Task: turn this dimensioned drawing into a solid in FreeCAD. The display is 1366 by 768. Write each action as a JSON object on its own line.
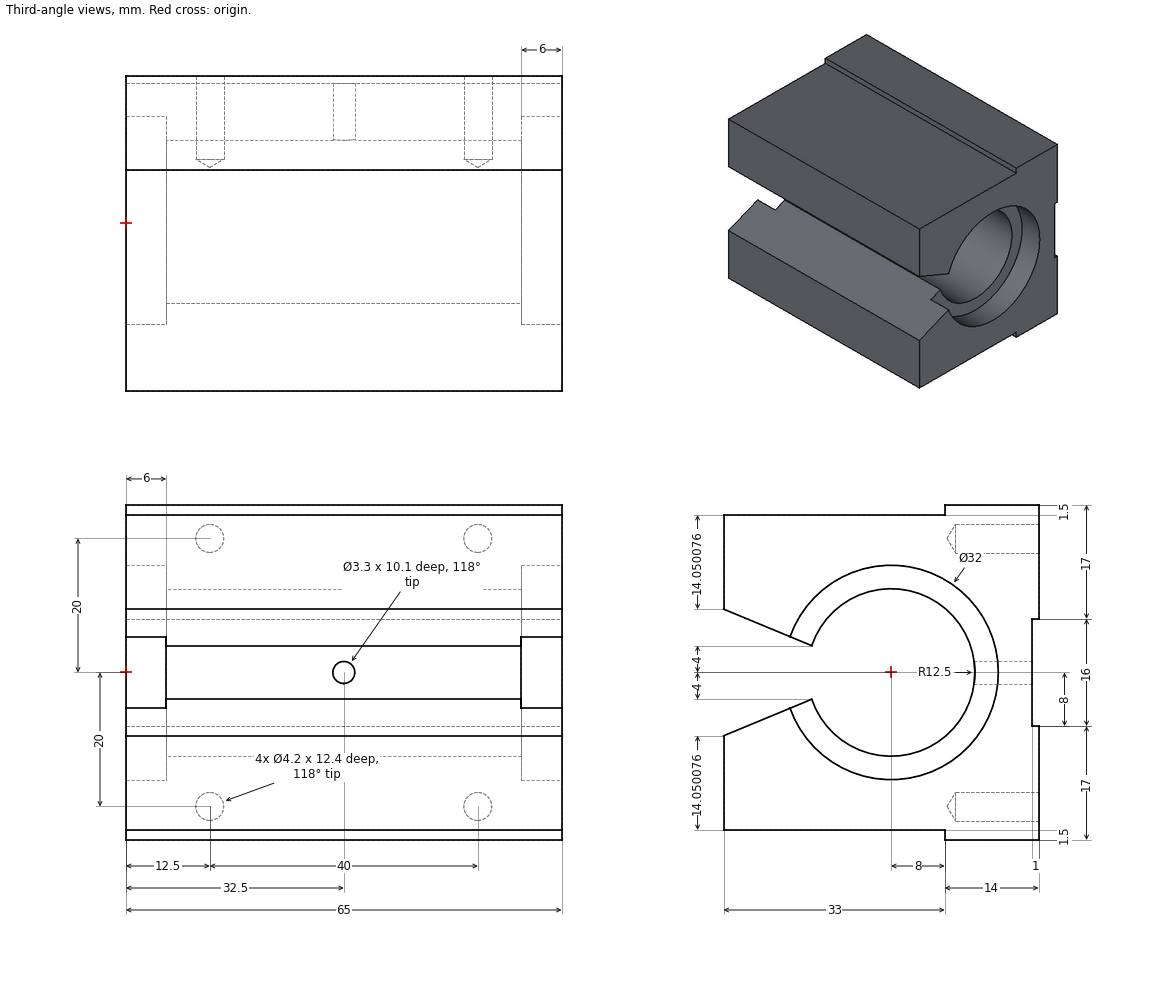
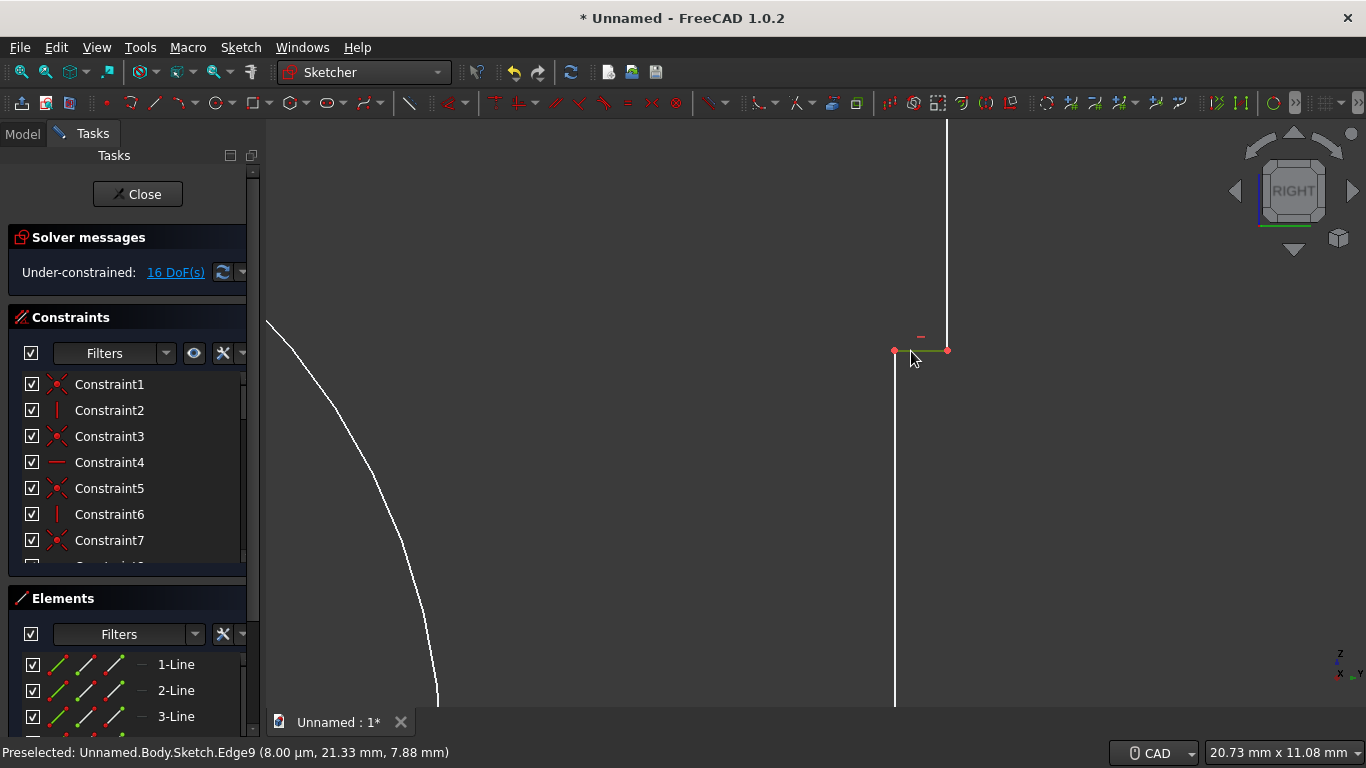
{"action": "key", "text": "l"}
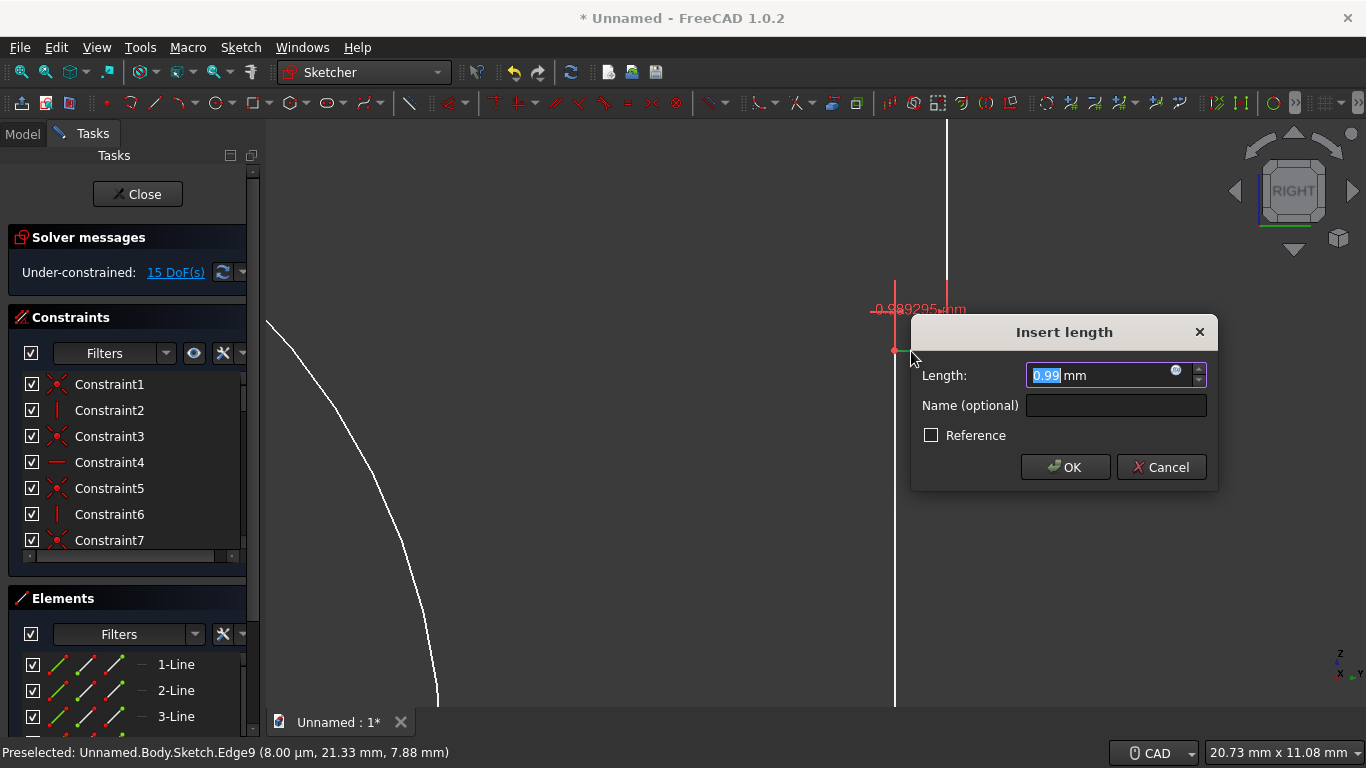
{"action": "type", "text": "1"}
{"action": "key", "text": "Return"}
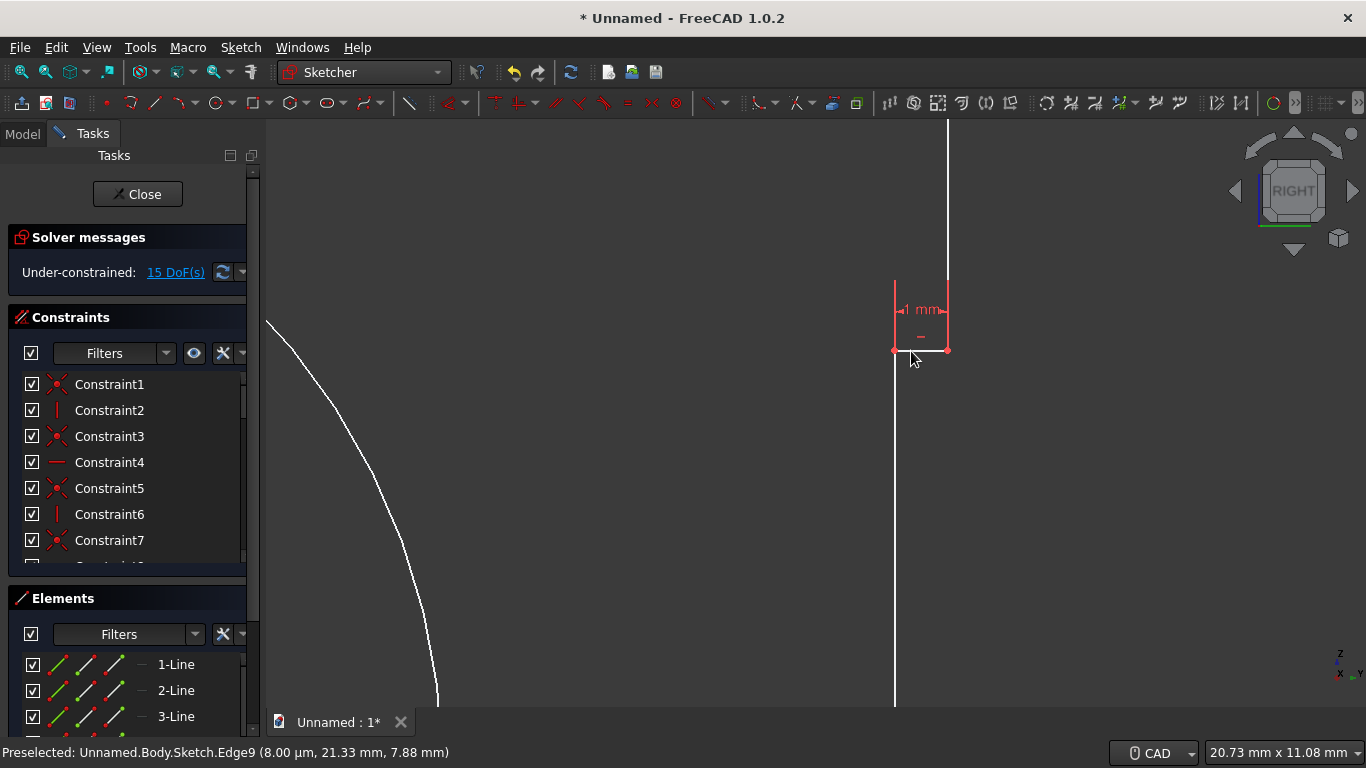
{"action": "scroll", "coordinate": [912, 357], "scroll_direction": "down", "scroll_amount": 10}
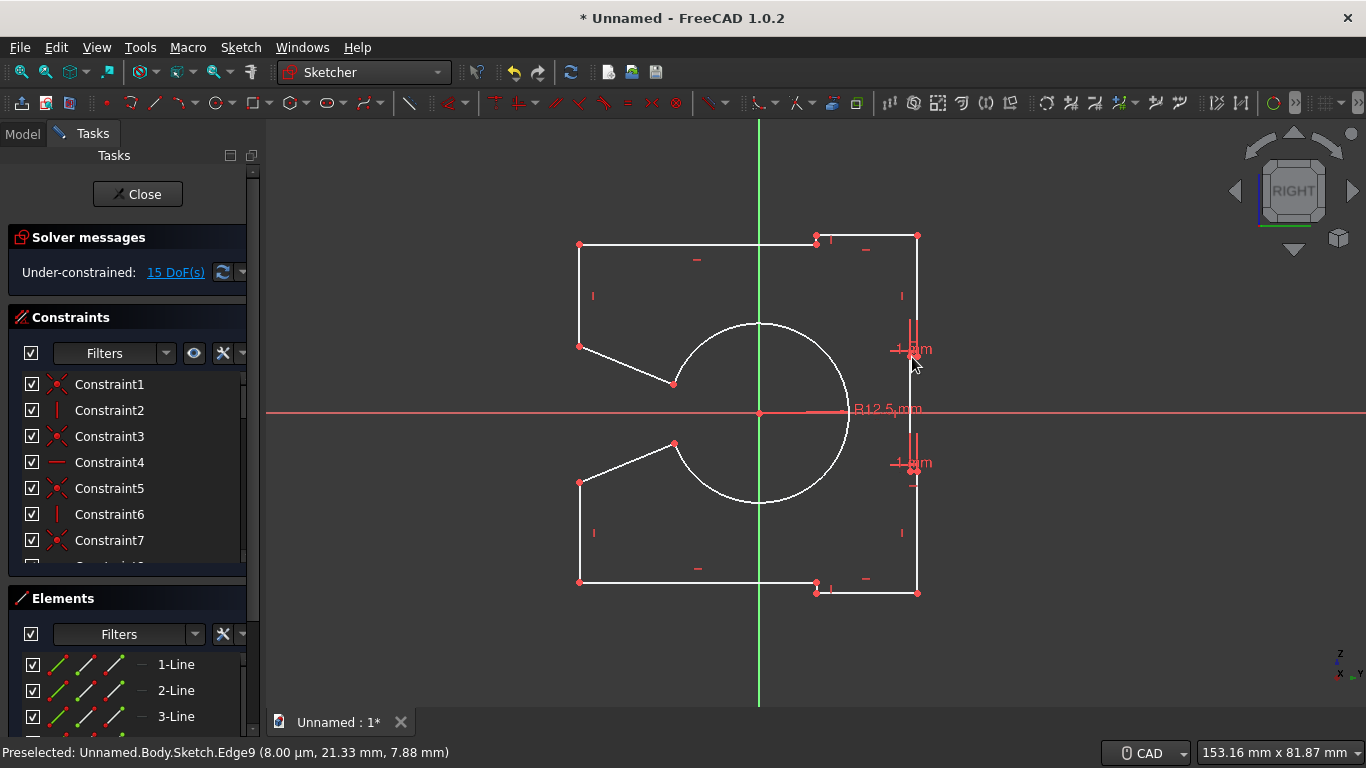
{"action": "left_click", "coordinate": [651, 583]}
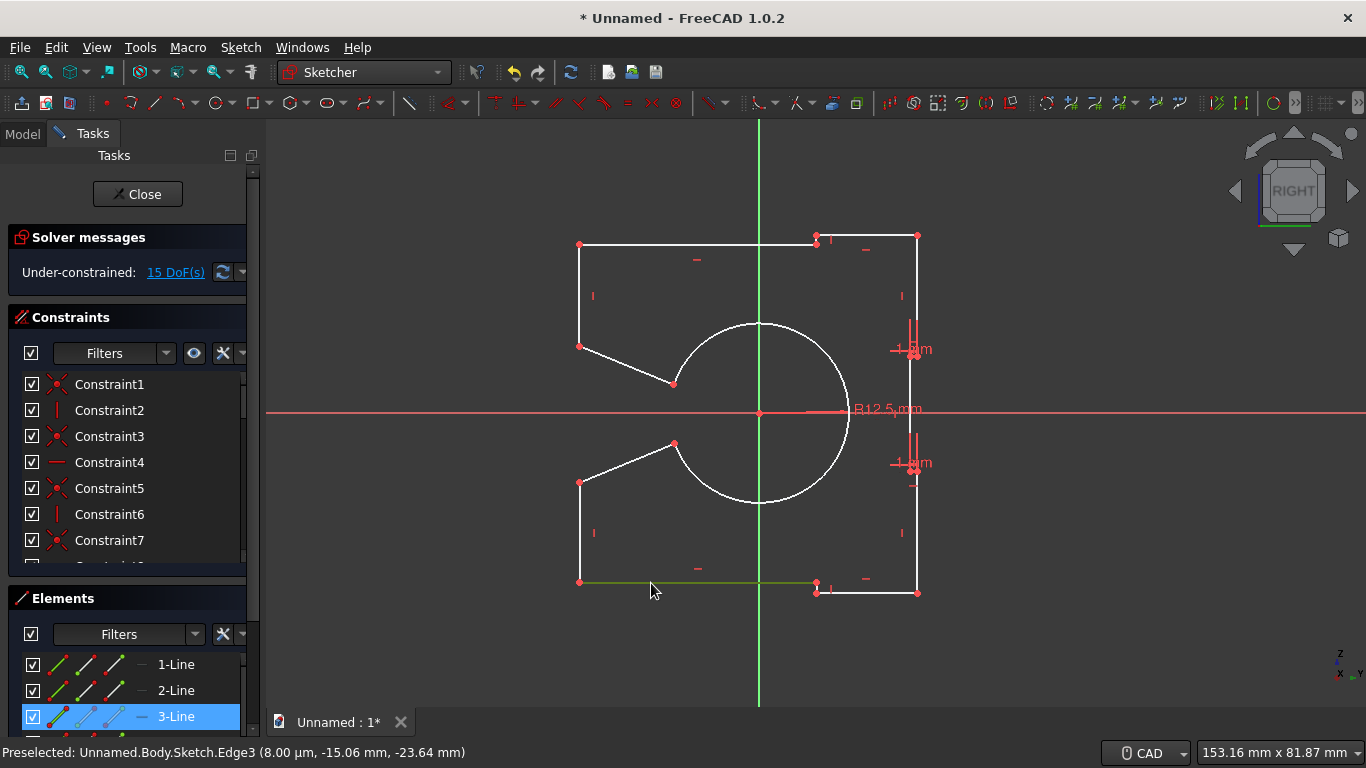
{"action": "key", "text": "l"}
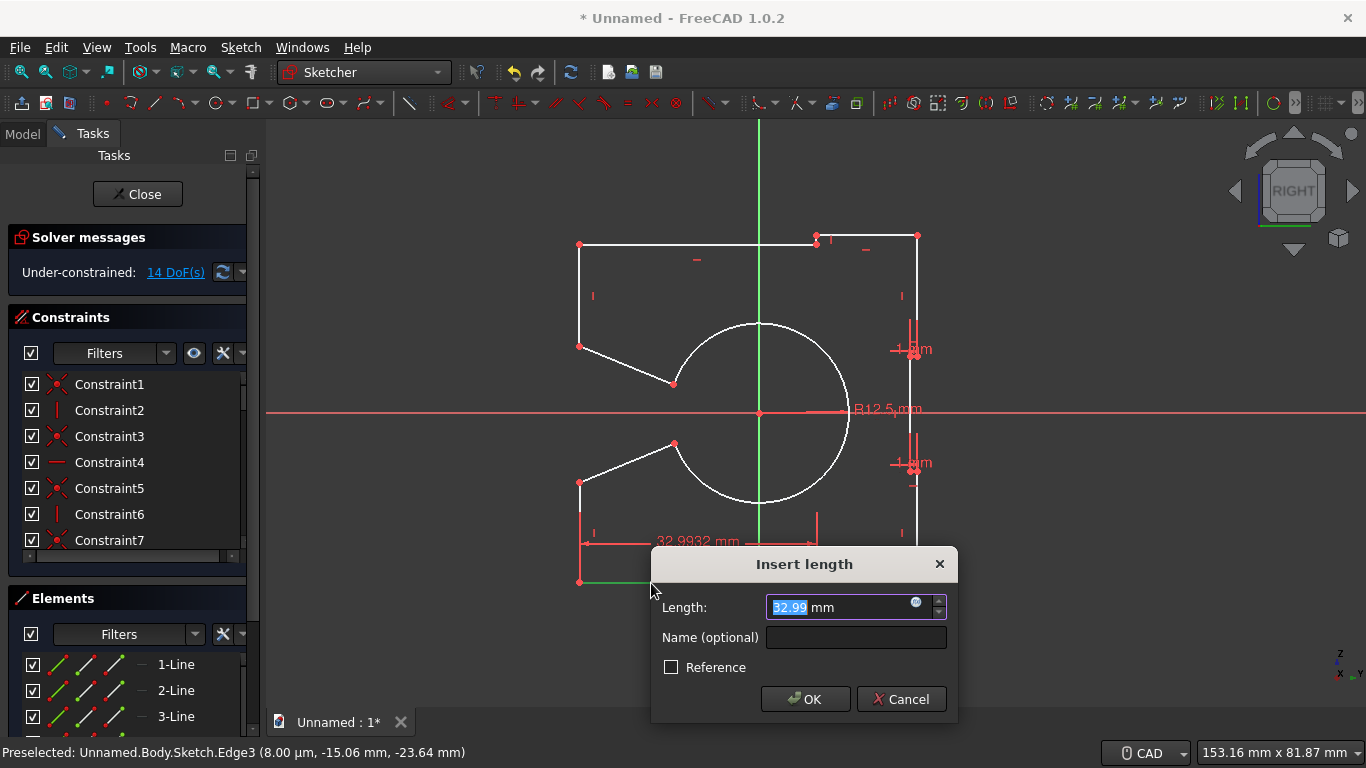
{"action": "type", "text": "33"}
{"action": "key", "text": "Return"}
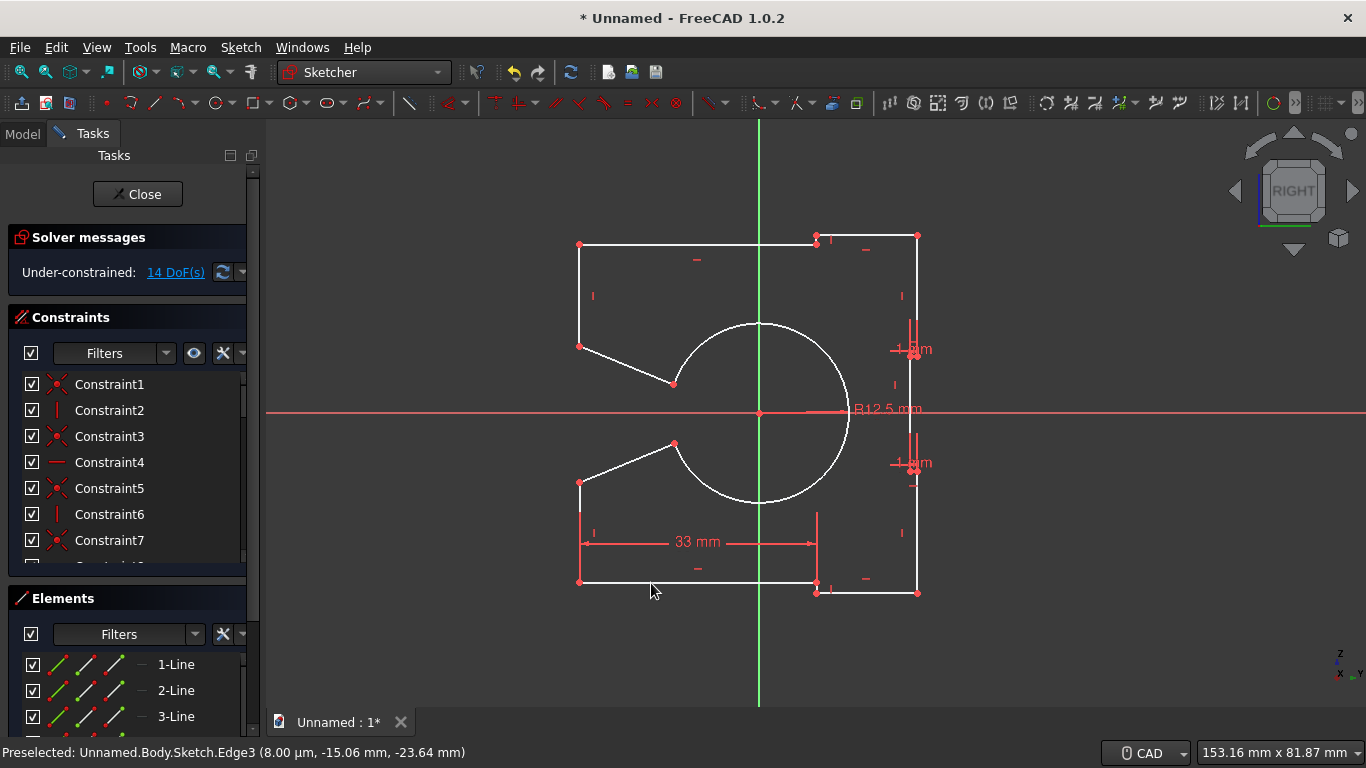
{"action": "left_click", "coordinate": [847, 593]}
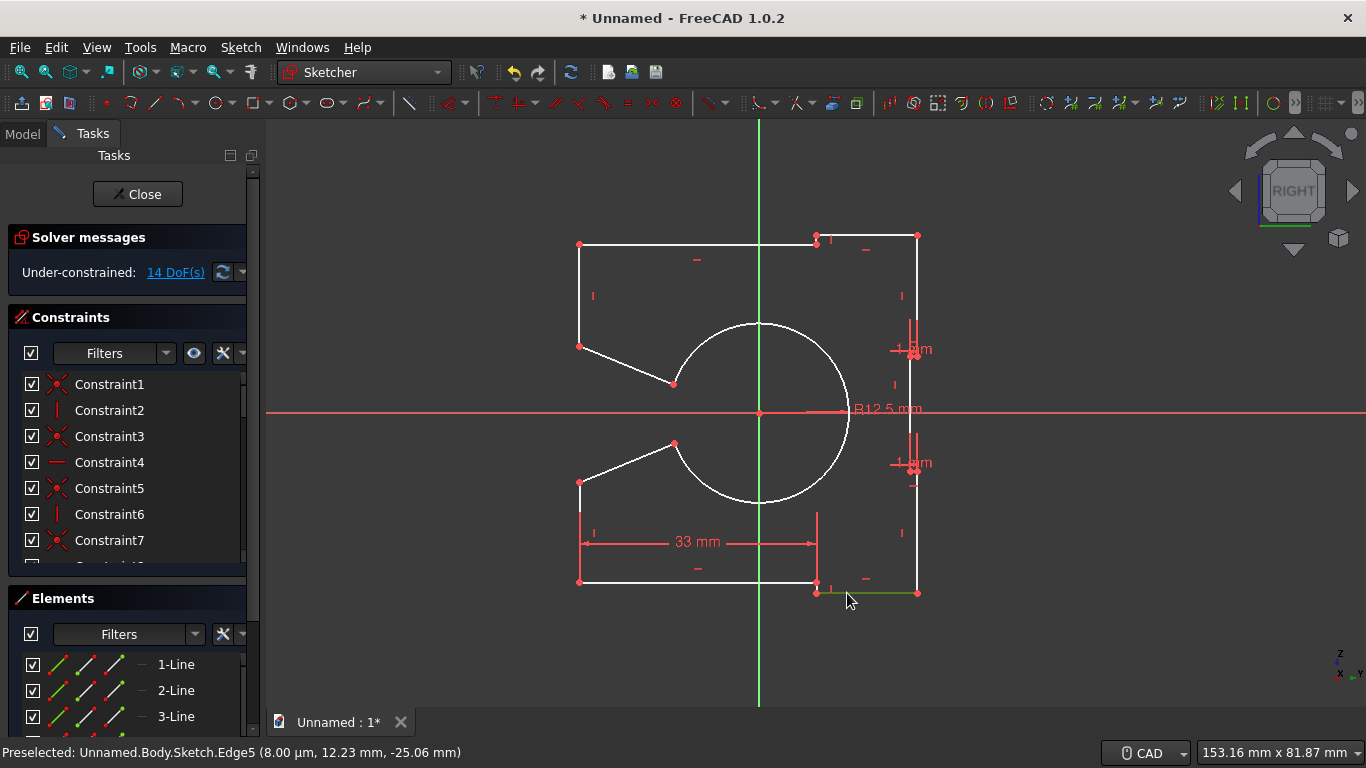
{"action": "key", "text": "l"}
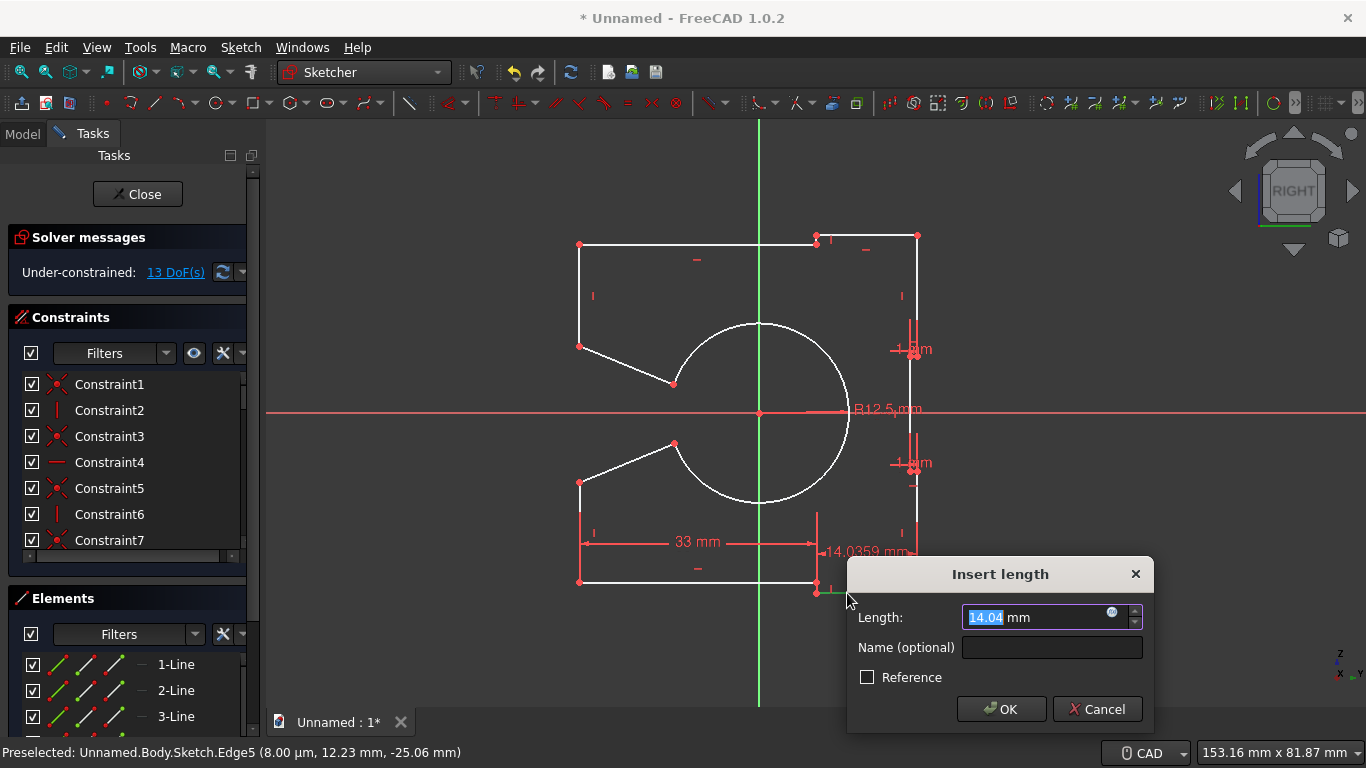
{"action": "type", "text": "14"}
{"action": "key", "text": "Return"}